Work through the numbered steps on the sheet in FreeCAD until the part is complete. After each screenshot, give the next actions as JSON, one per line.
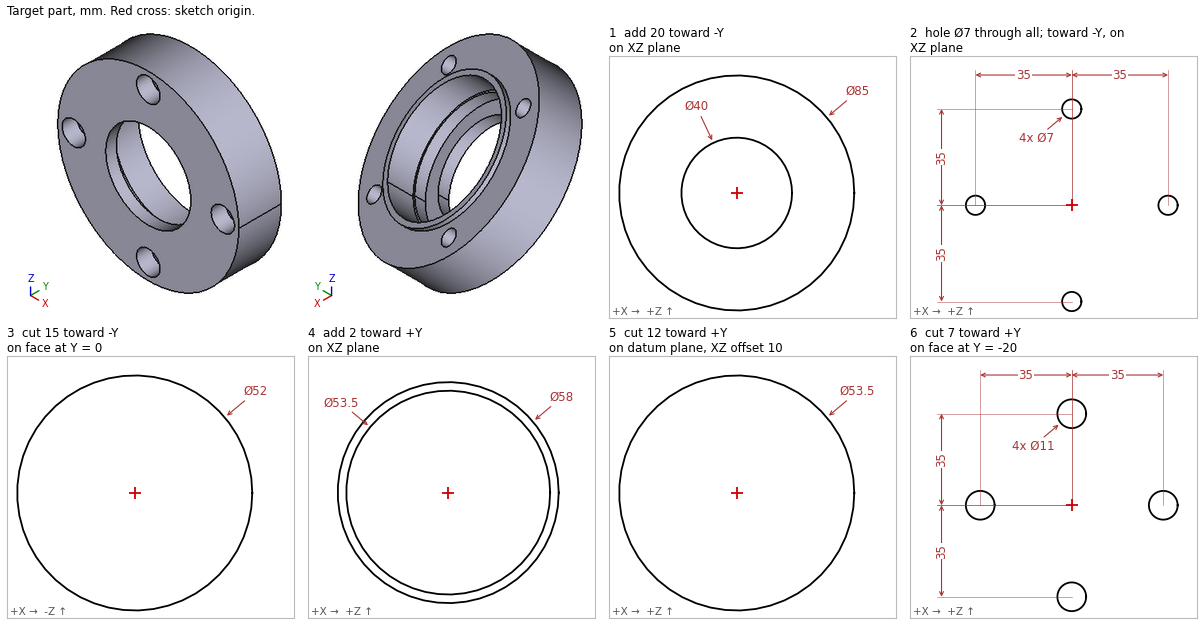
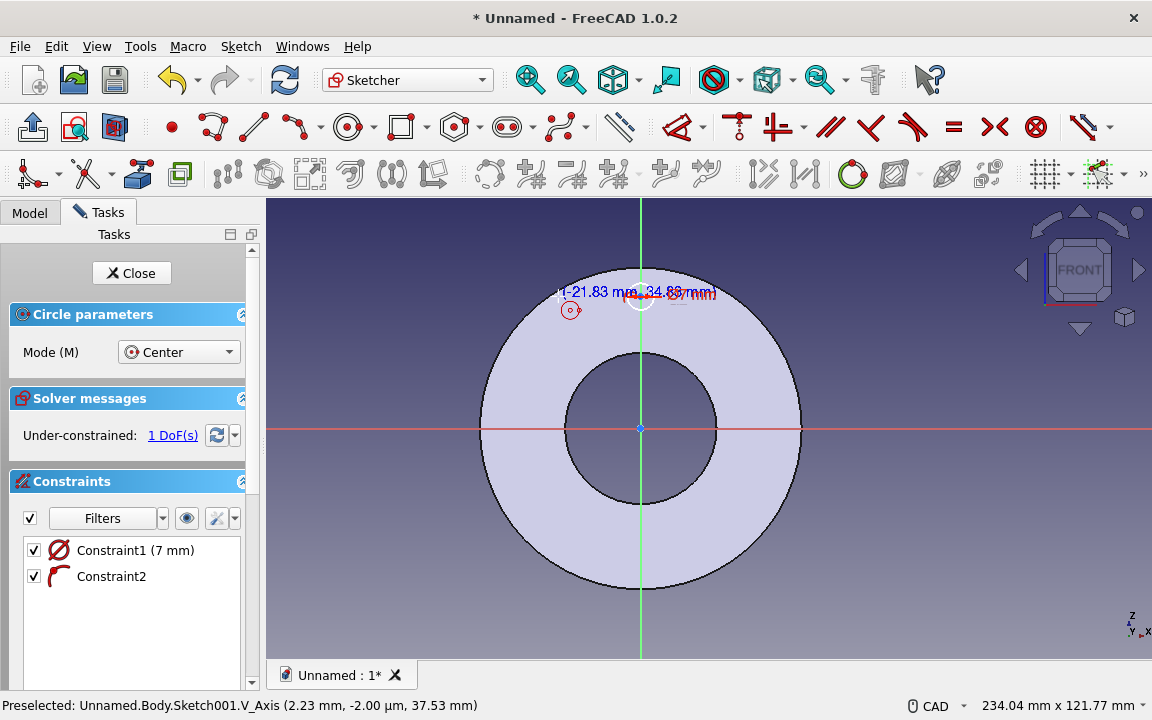
{"action": "scroll", "coordinate": [641, 561], "scroll_direction": "up", "scroll_amount": 3}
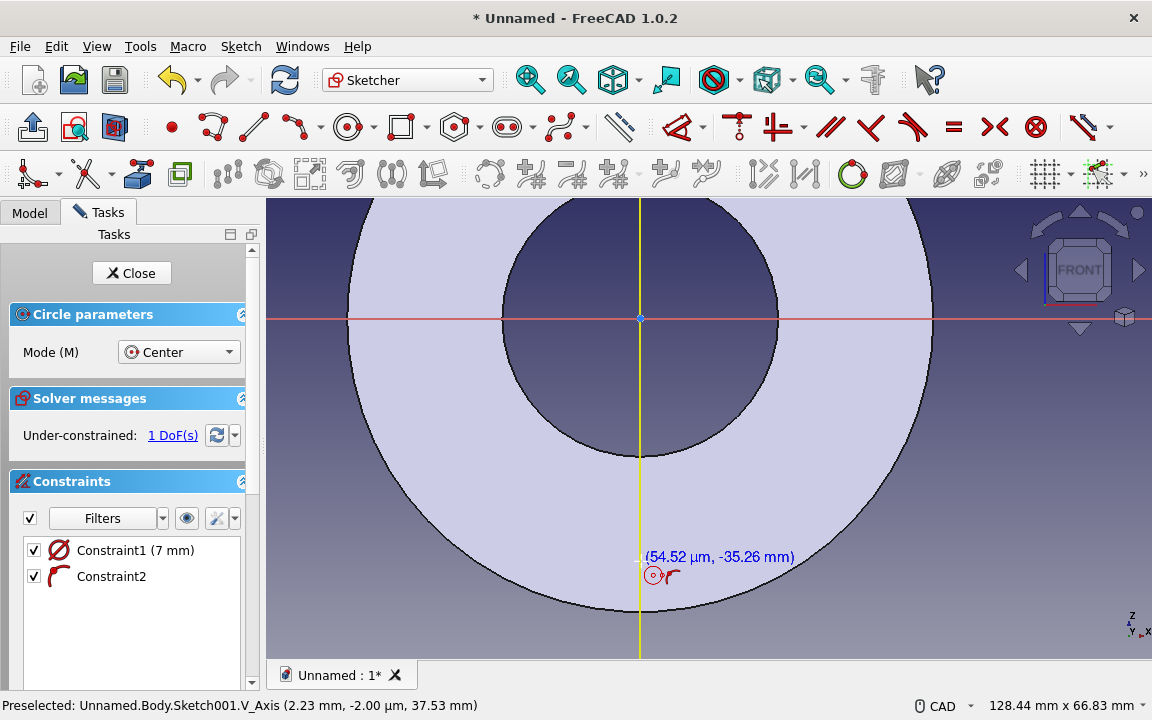
{"action": "left_click", "coordinate": [640, 560]}
{"action": "mouse_move", "coordinate": [657, 543]}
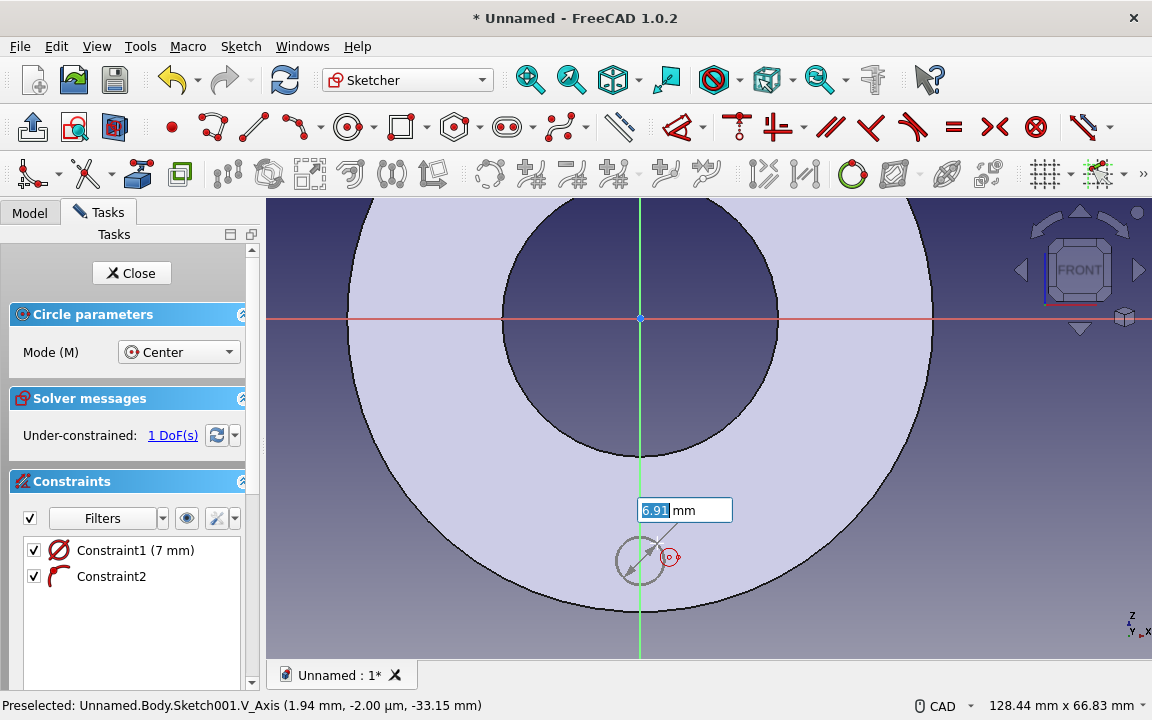
{"action": "type", "text": "7"}
{"action": "key", "text": "Return"}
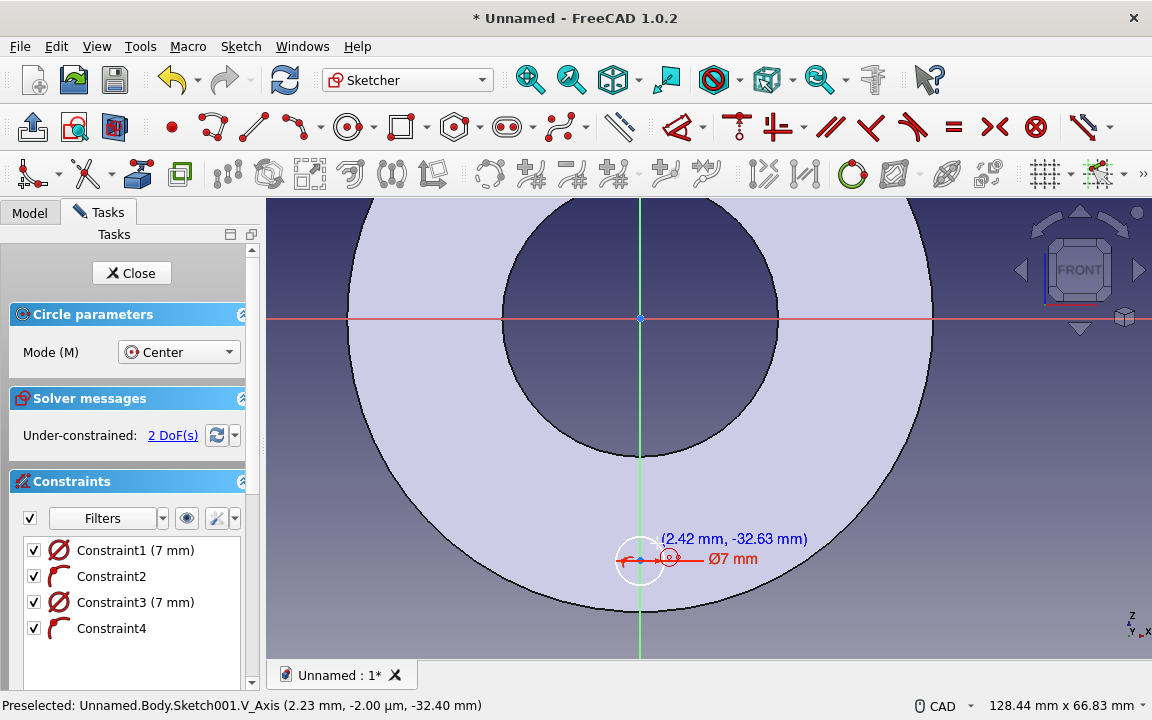
{"action": "left_click", "coordinate": [399, 319]}
{"action": "mouse_move", "coordinate": [416, 302]}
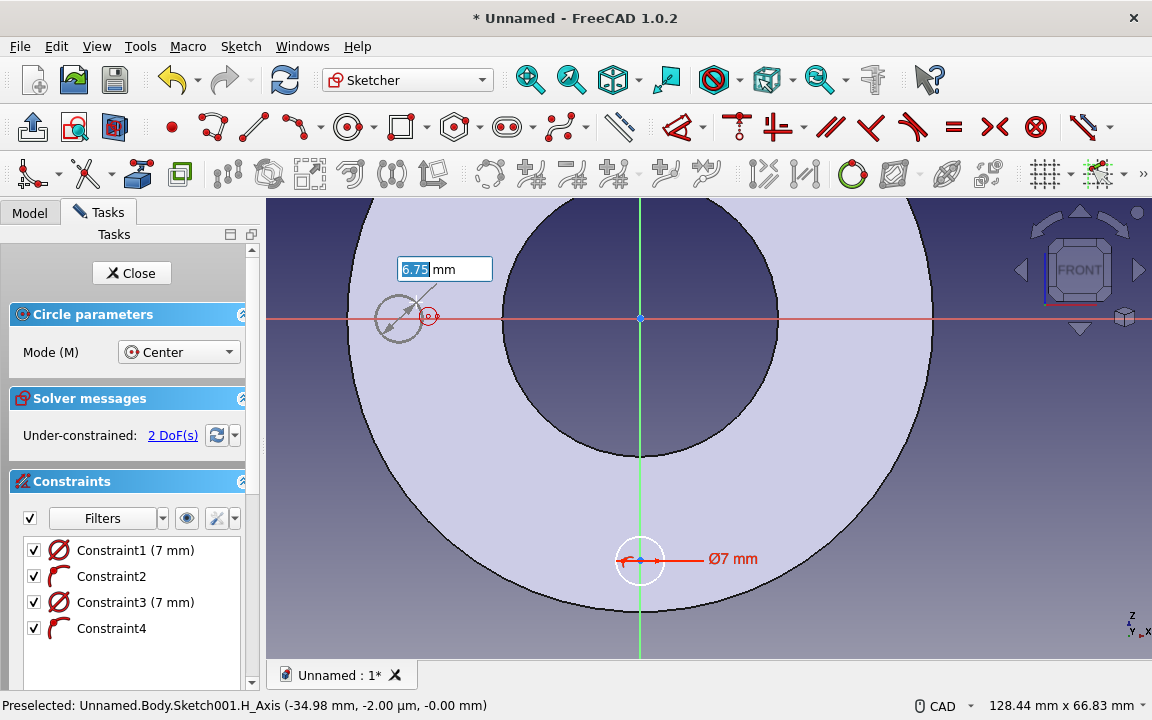
{"action": "type", "text": "7"}
{"action": "key", "text": "Return"}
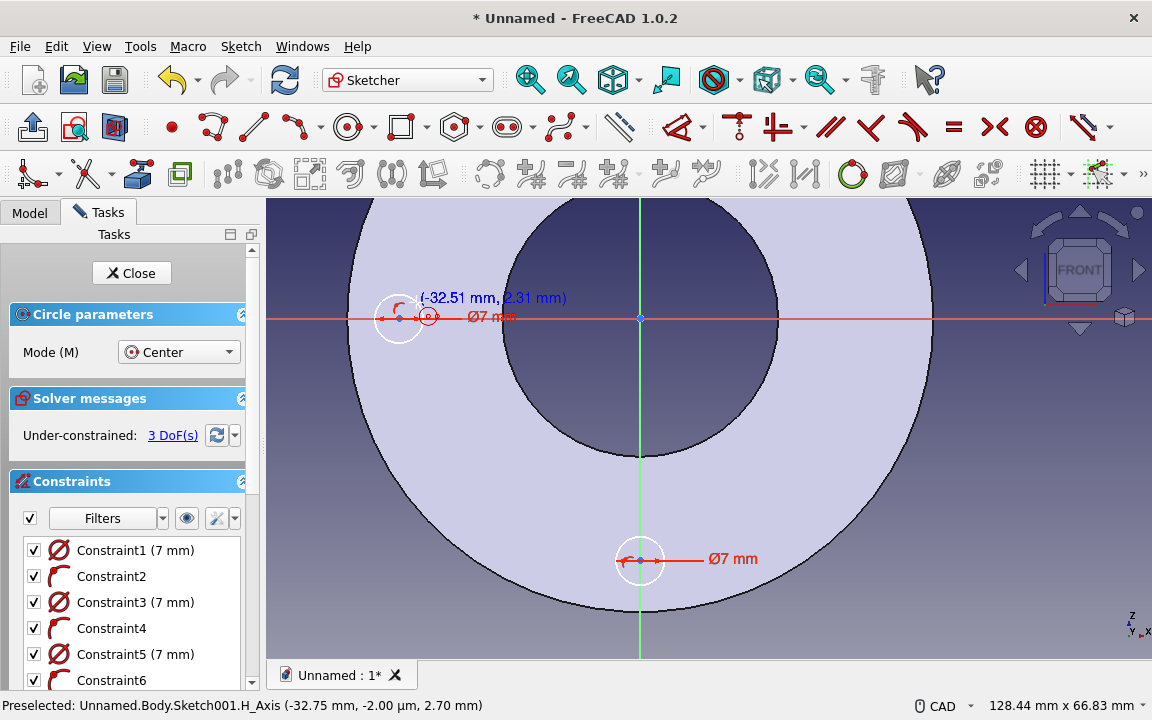
{"action": "left_click", "coordinate": [882, 319]}
{"action": "mouse_move", "coordinate": [899, 302]}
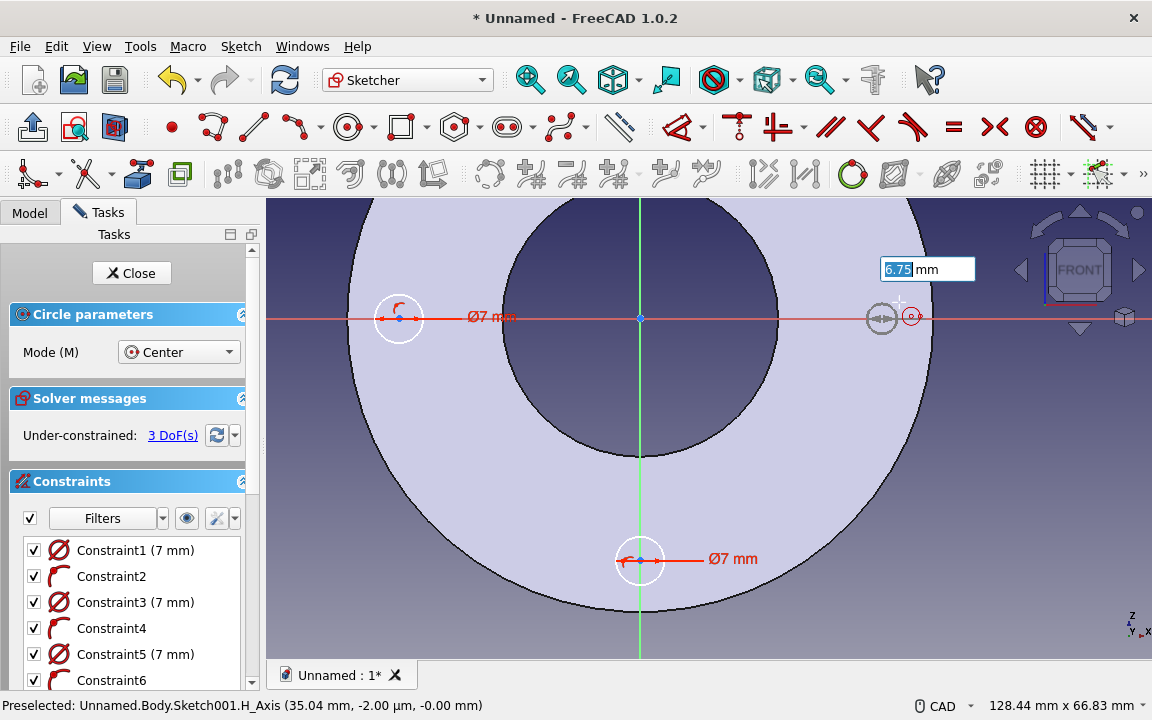
{"action": "type", "text": "7"}
{"action": "key", "text": "Return"}
{"action": "key", "text": "Escape"}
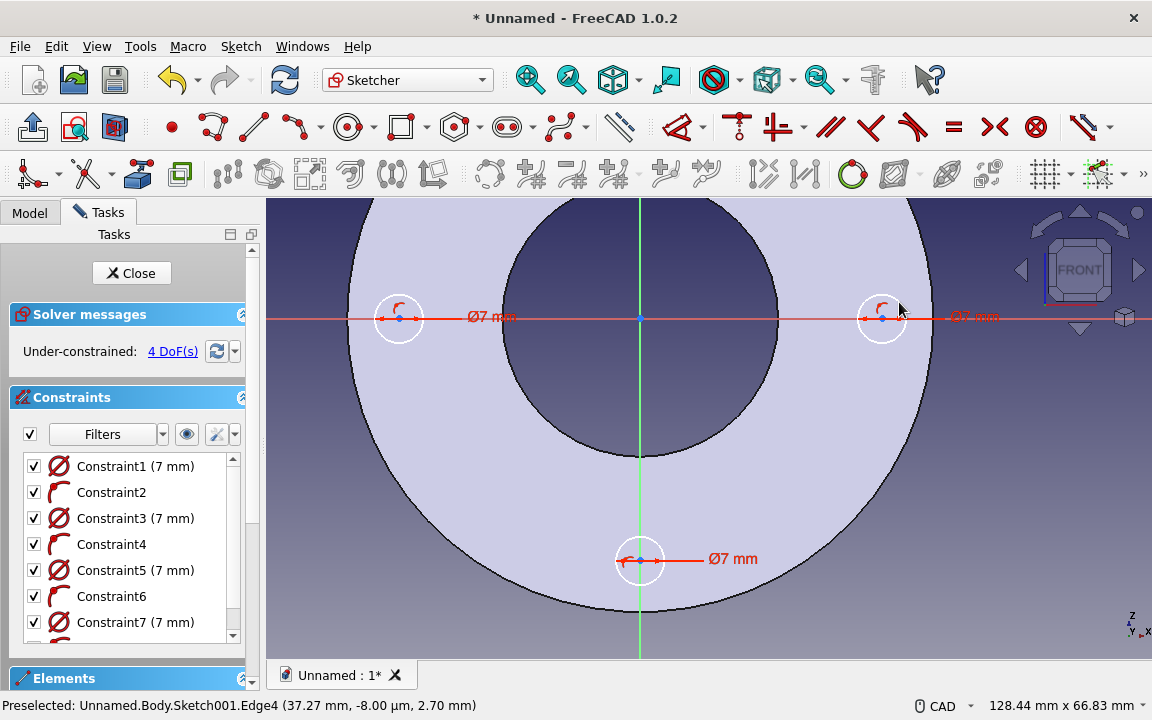
{"action": "scroll", "coordinate": [641, 562], "scroll_direction": "down", "scroll_amount": 3}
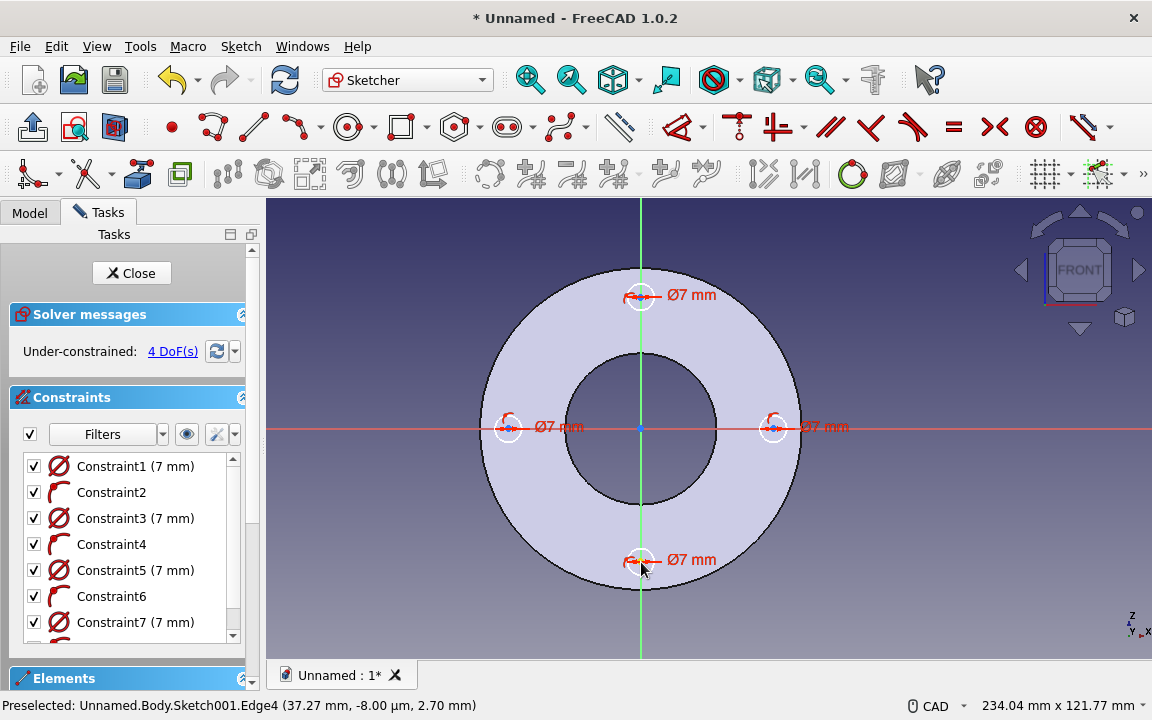
{"action": "left_click", "coordinate": [641, 297]}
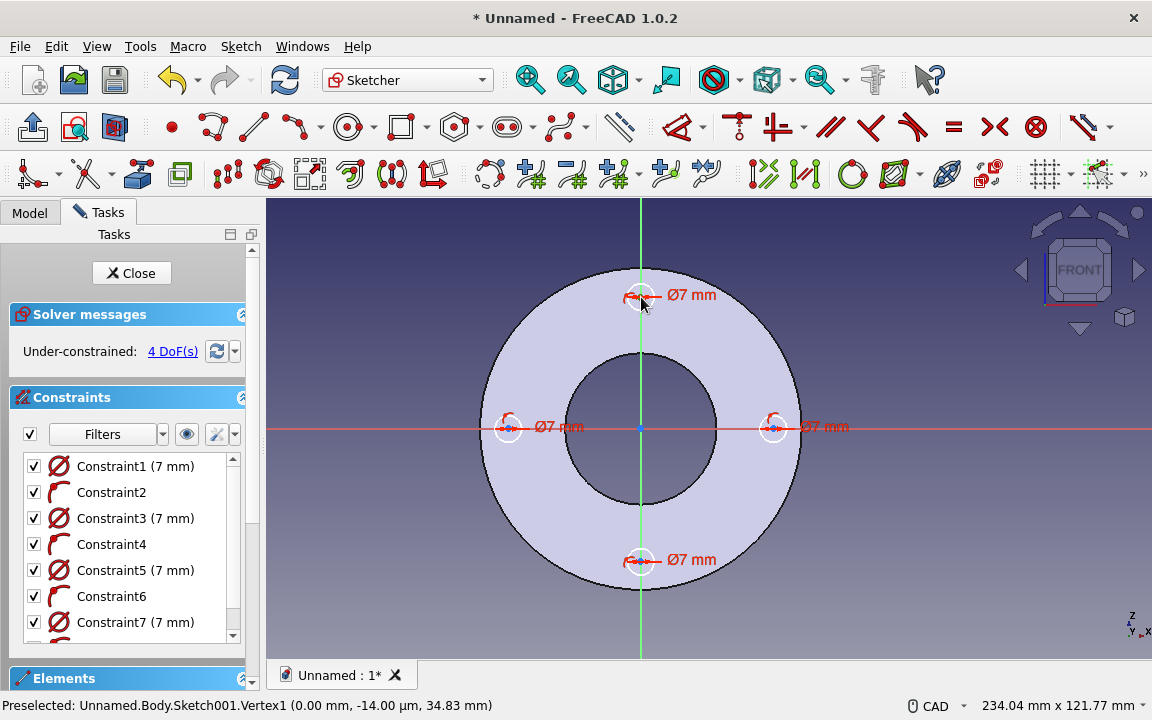
{"action": "key", "text": "i"}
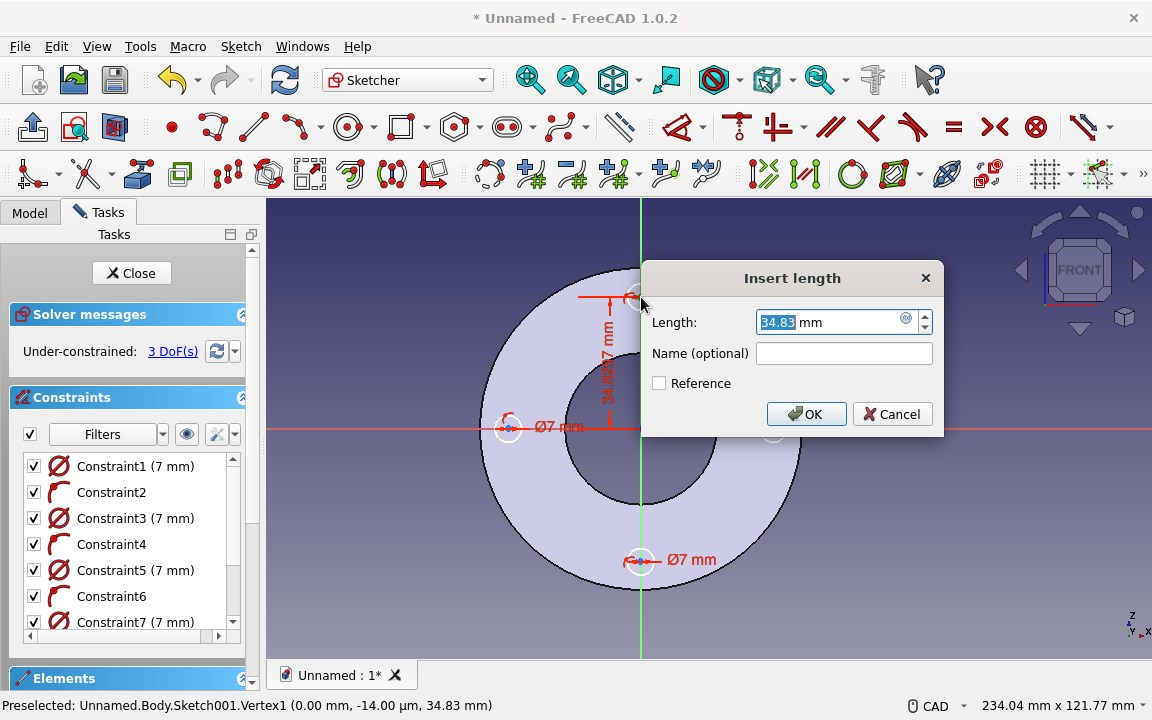
{"action": "type", "text": "35"}
{"action": "key", "text": "Return"}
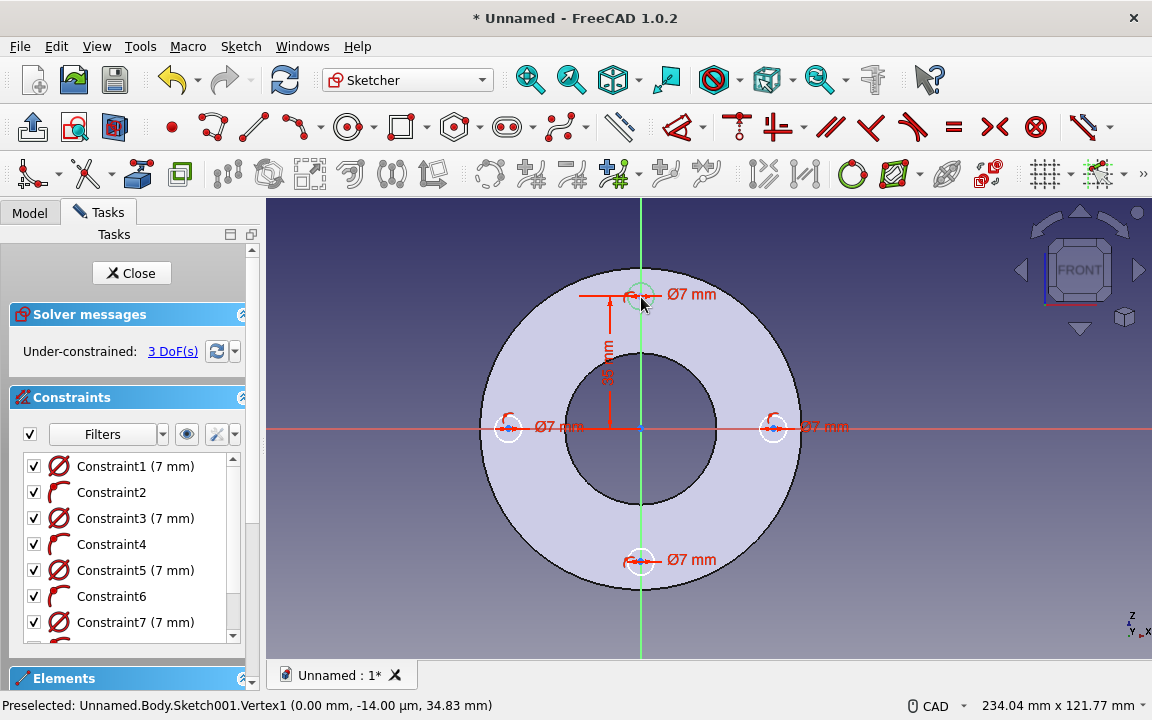
{"action": "left_click", "coordinate": [641, 562]}